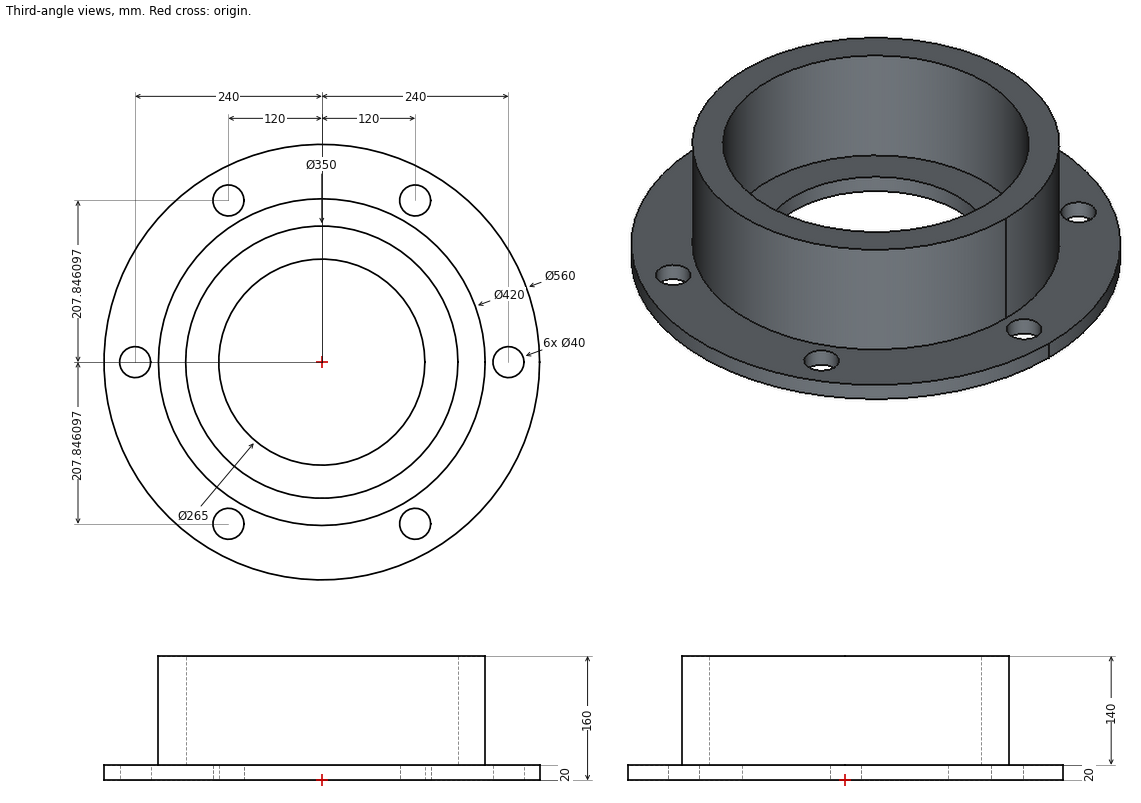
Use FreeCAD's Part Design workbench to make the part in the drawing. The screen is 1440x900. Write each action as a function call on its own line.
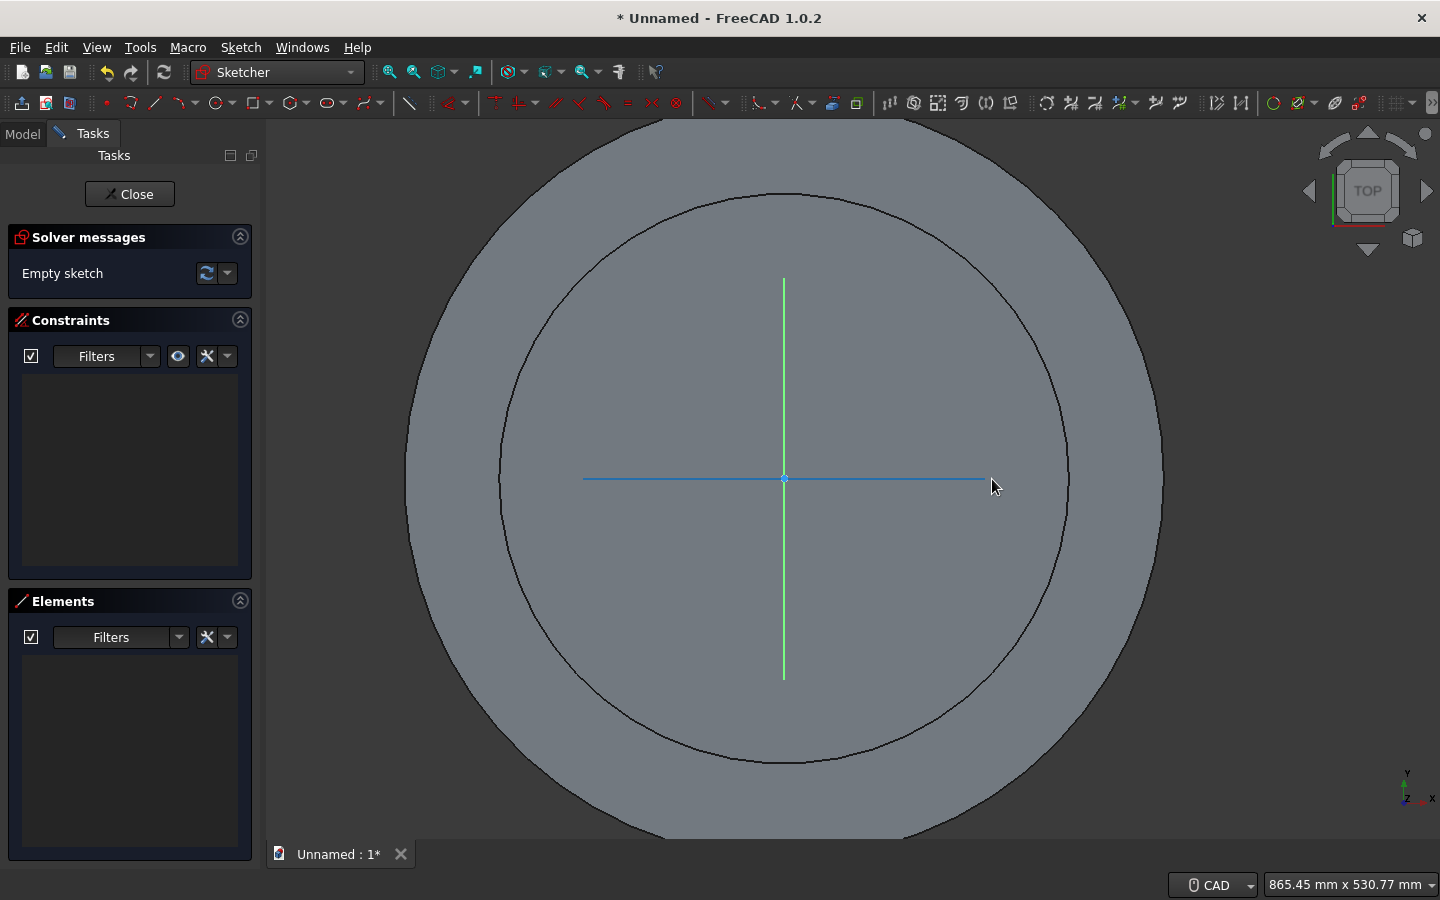
key(g)
key(c)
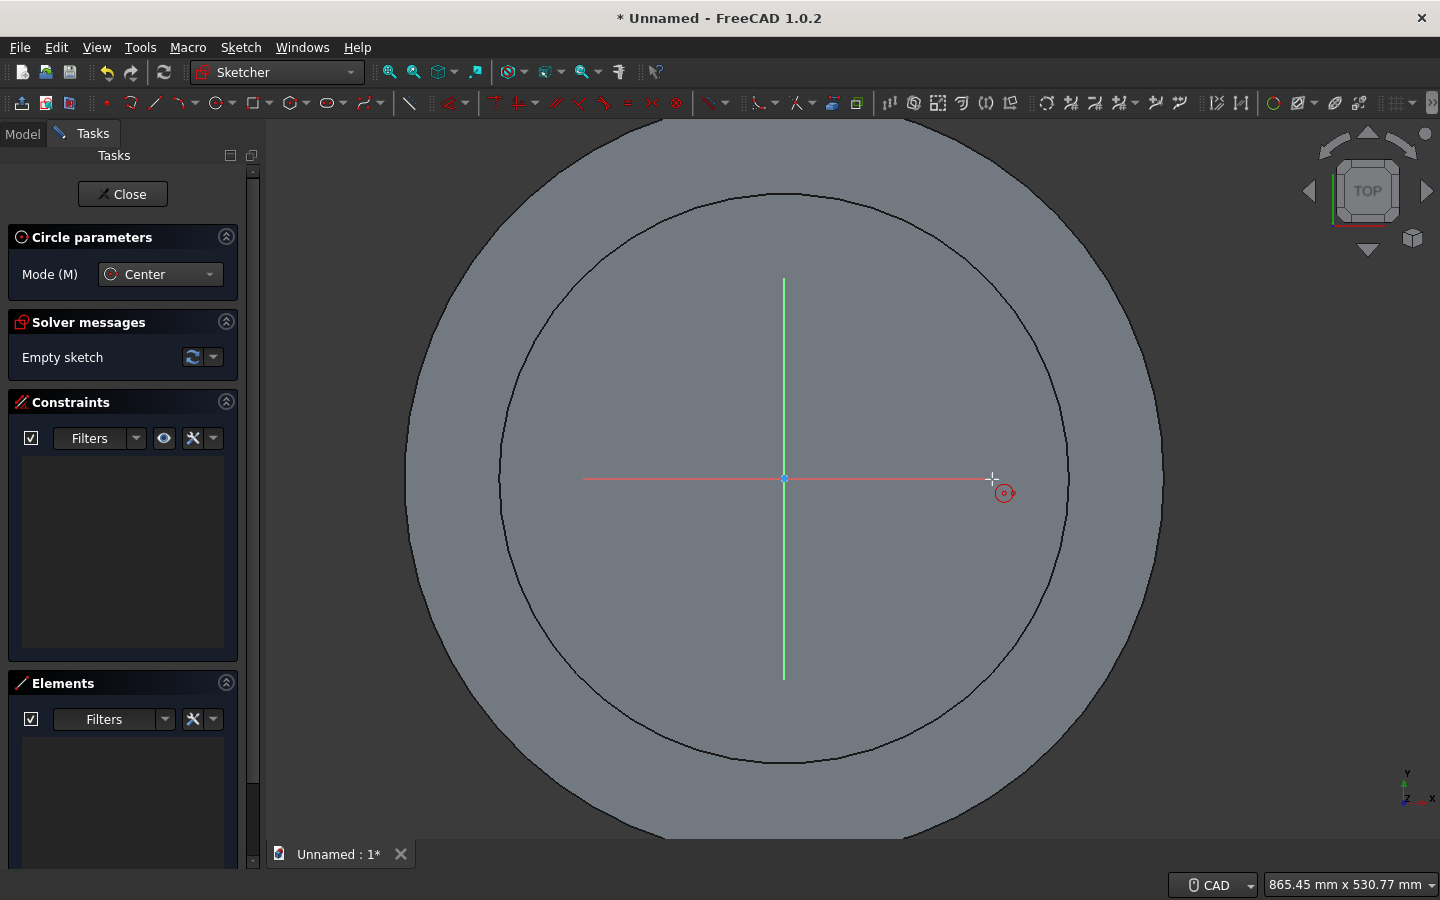
click(784, 479)
click(952, 311)
key(Escape)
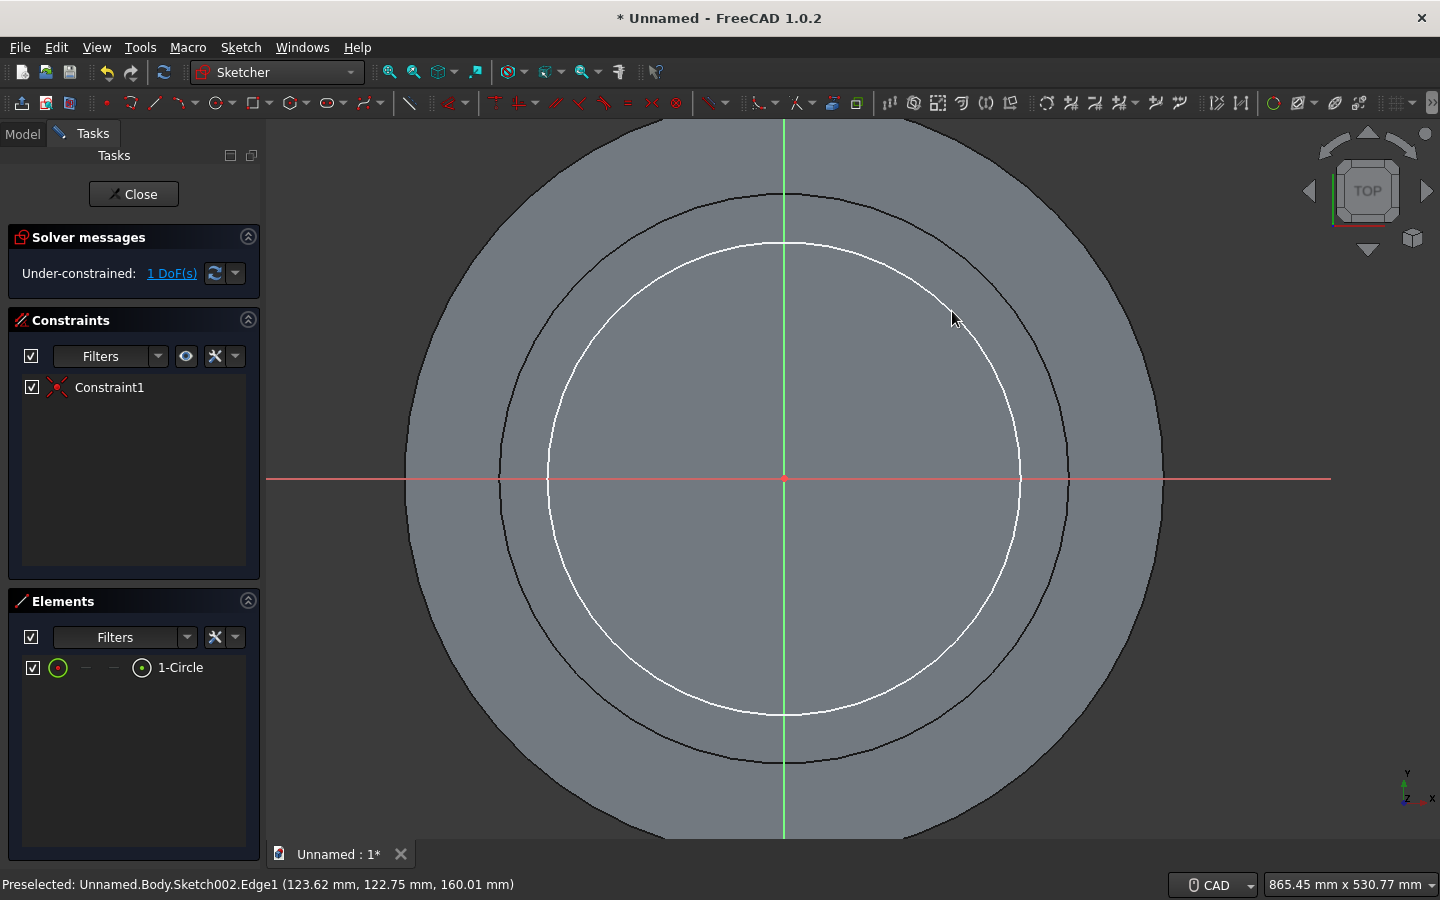
key(d)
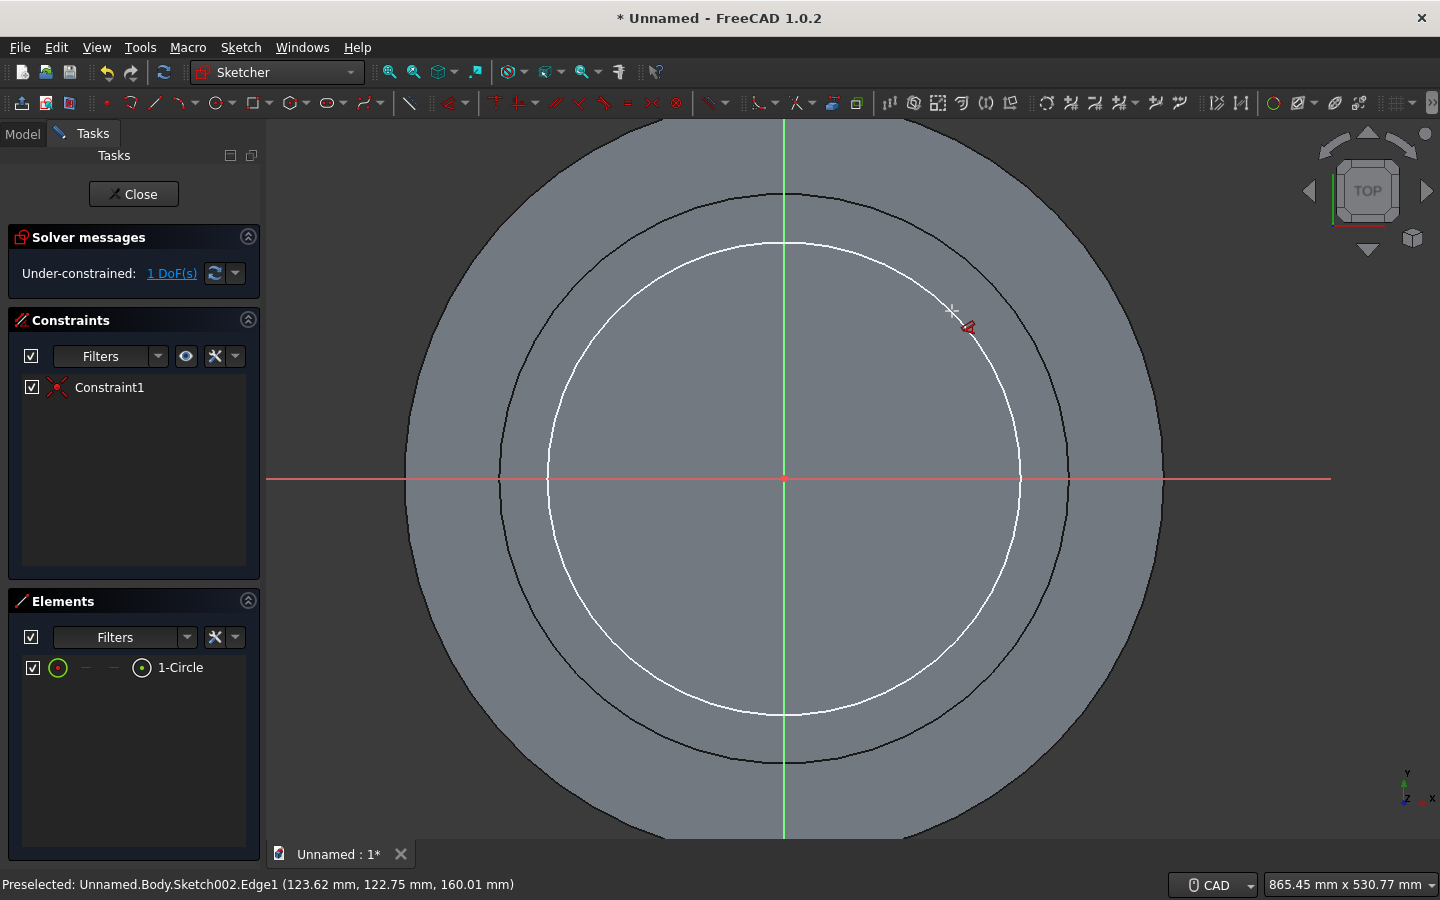
click(951, 311)
click(974, 288)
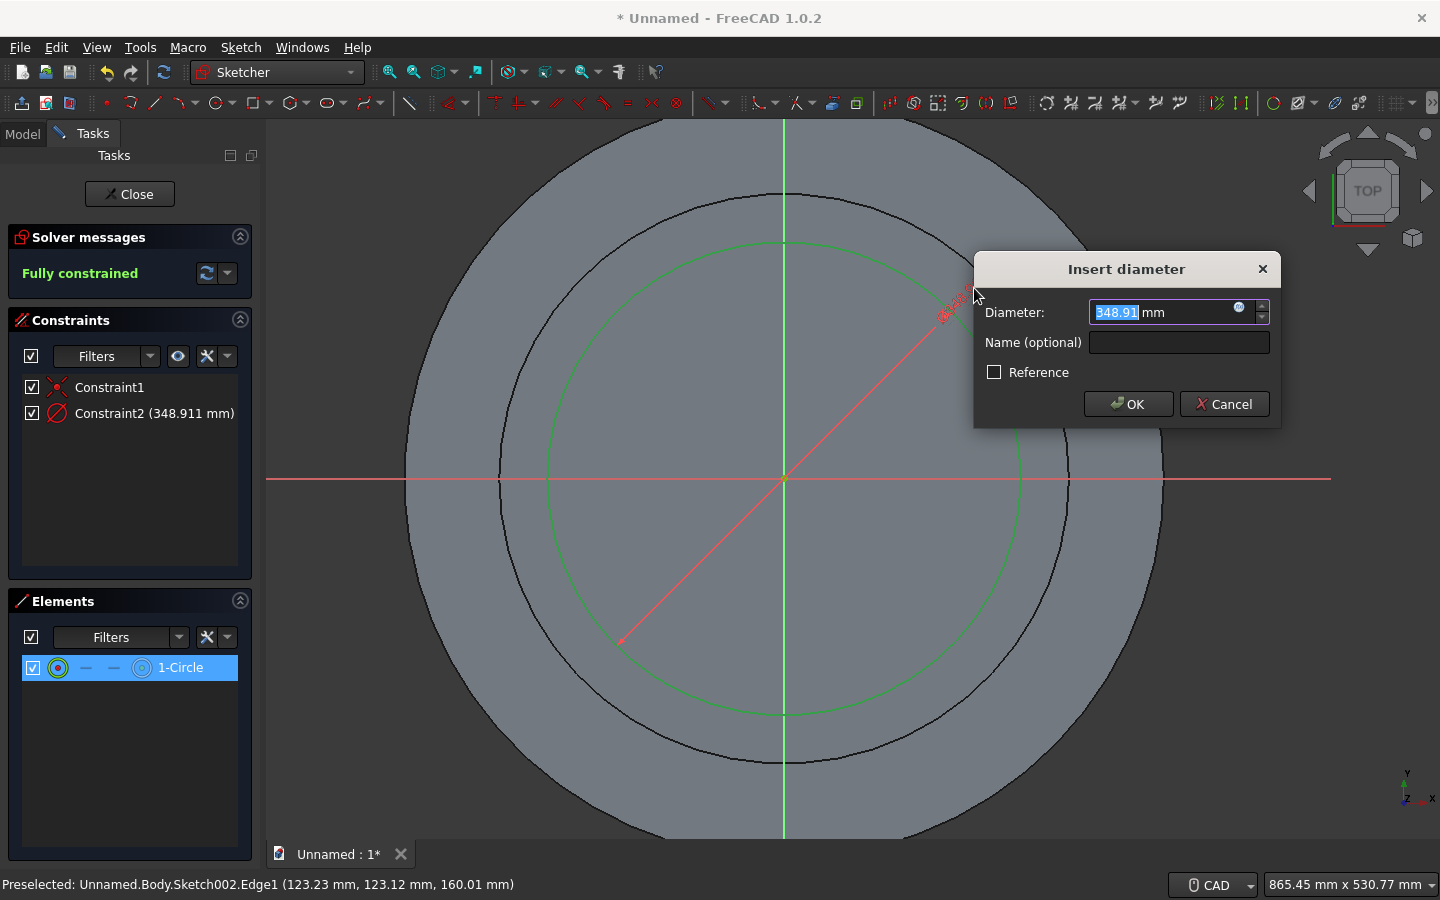
text(350)
key(Return)
key(Escape)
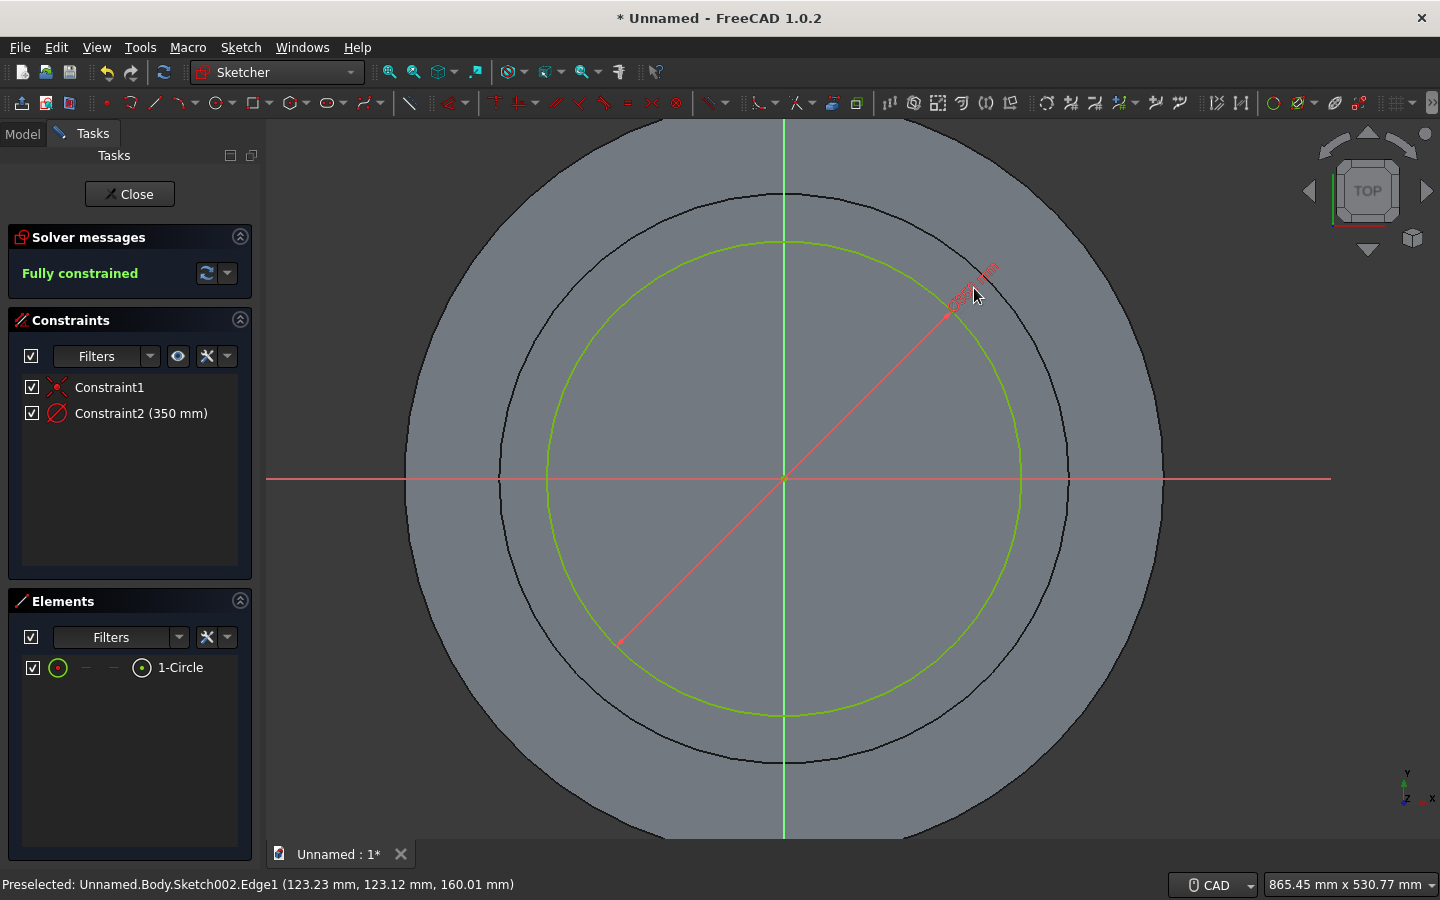
click(130, 194)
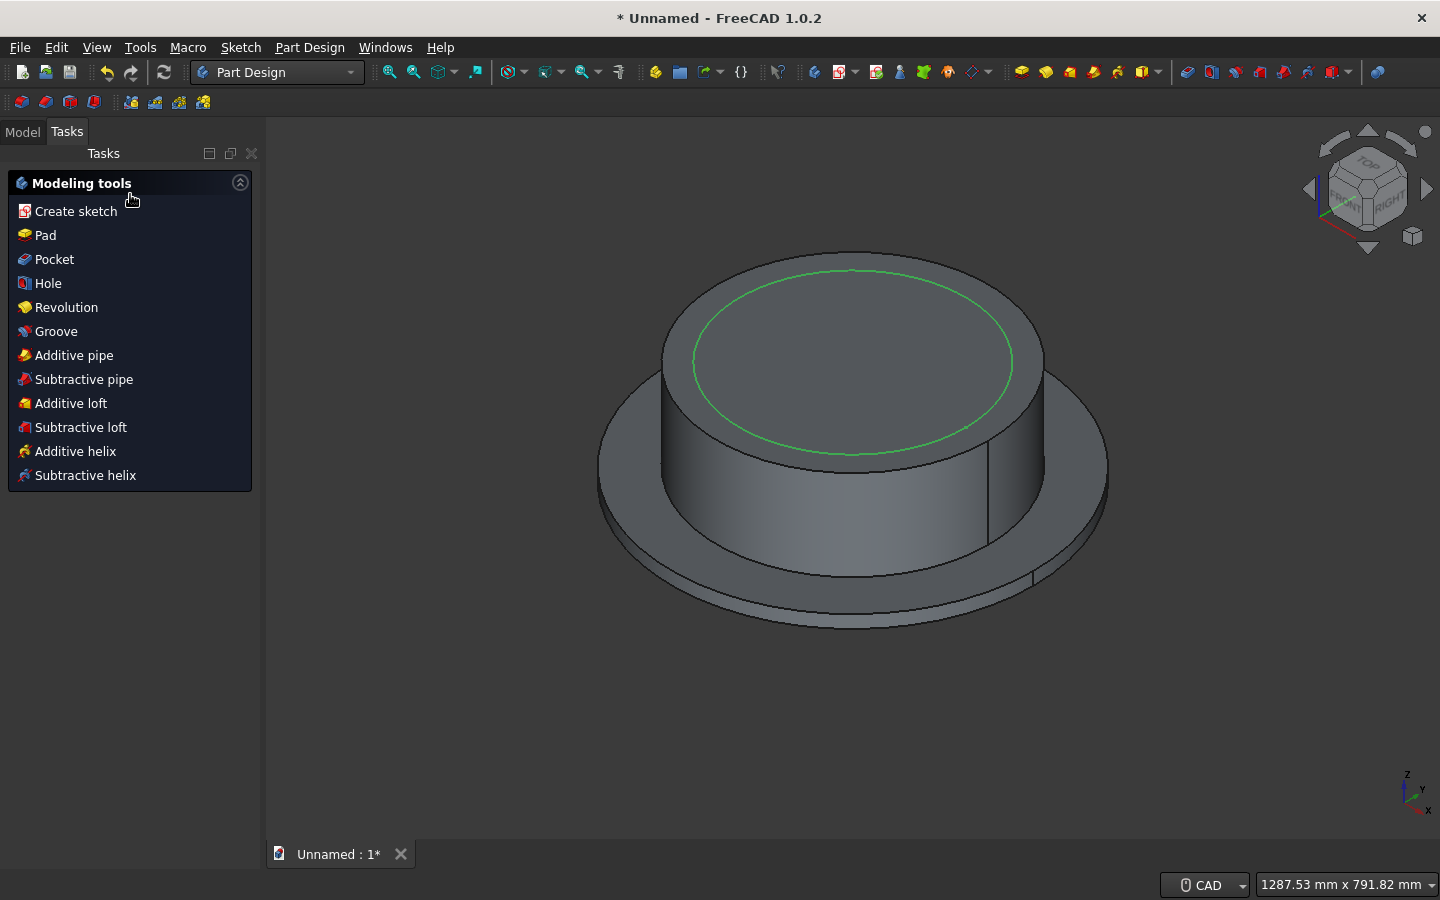
click(1188, 72)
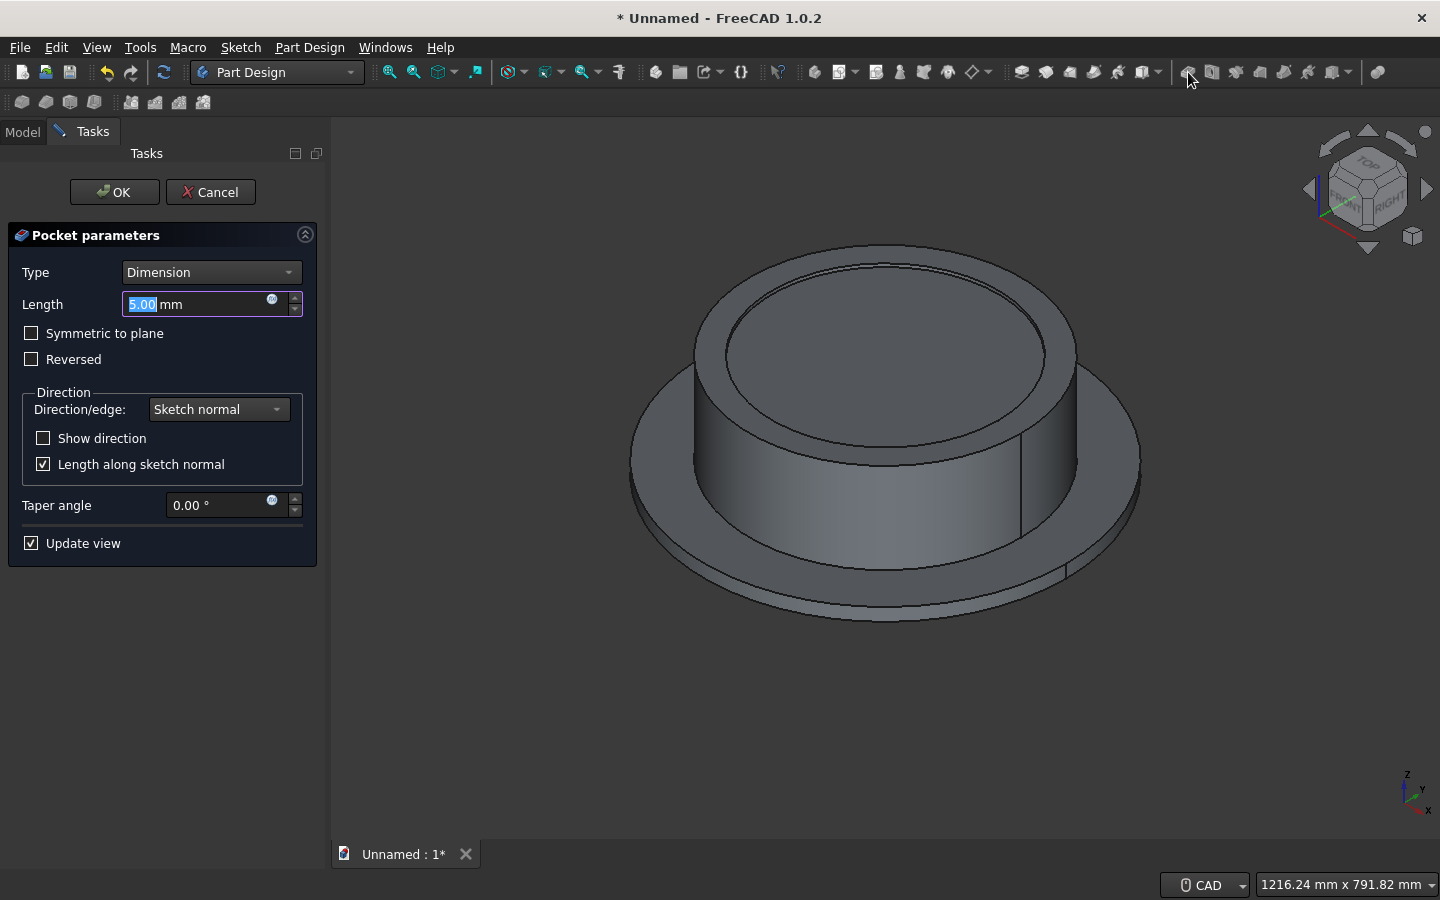
text(140)
key(Tab)